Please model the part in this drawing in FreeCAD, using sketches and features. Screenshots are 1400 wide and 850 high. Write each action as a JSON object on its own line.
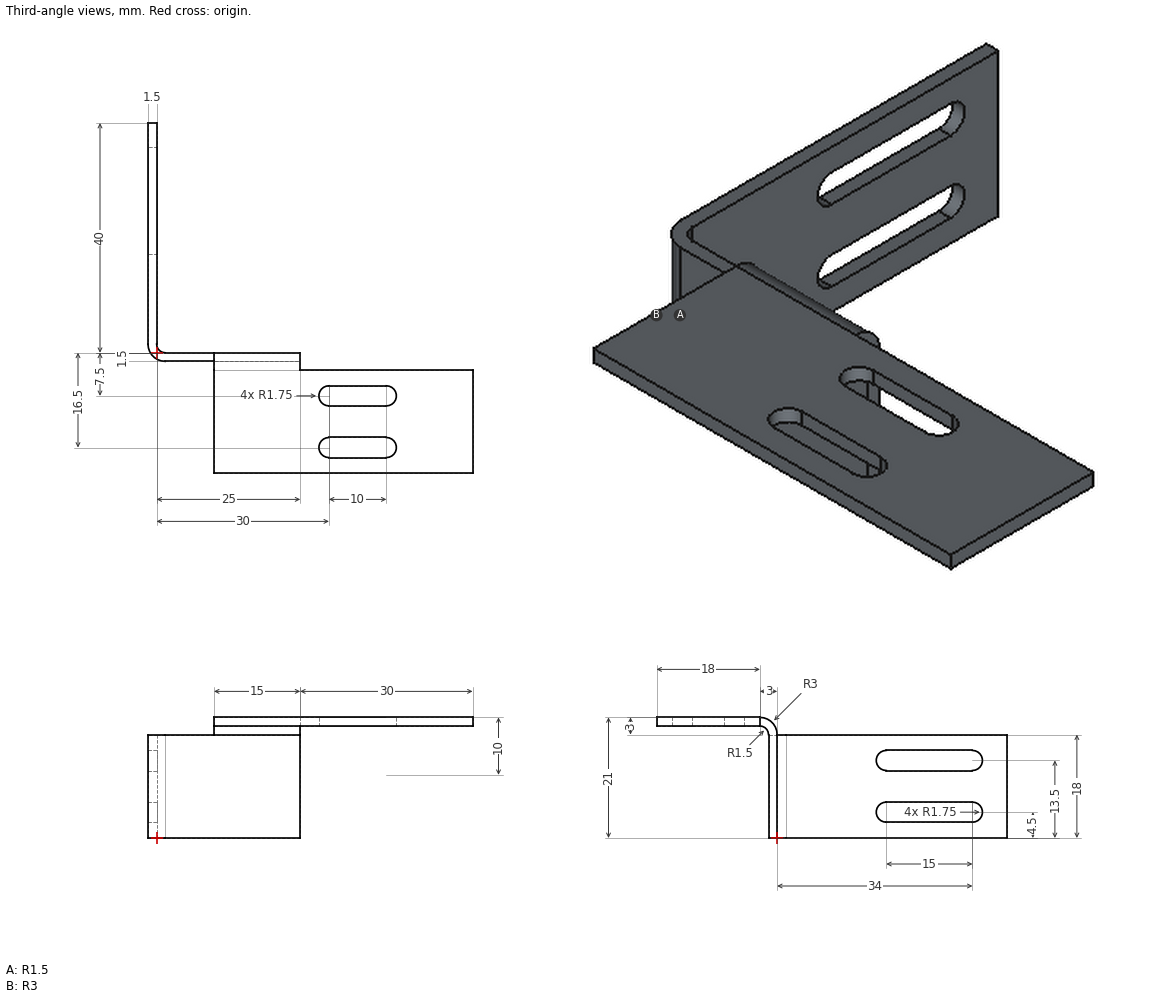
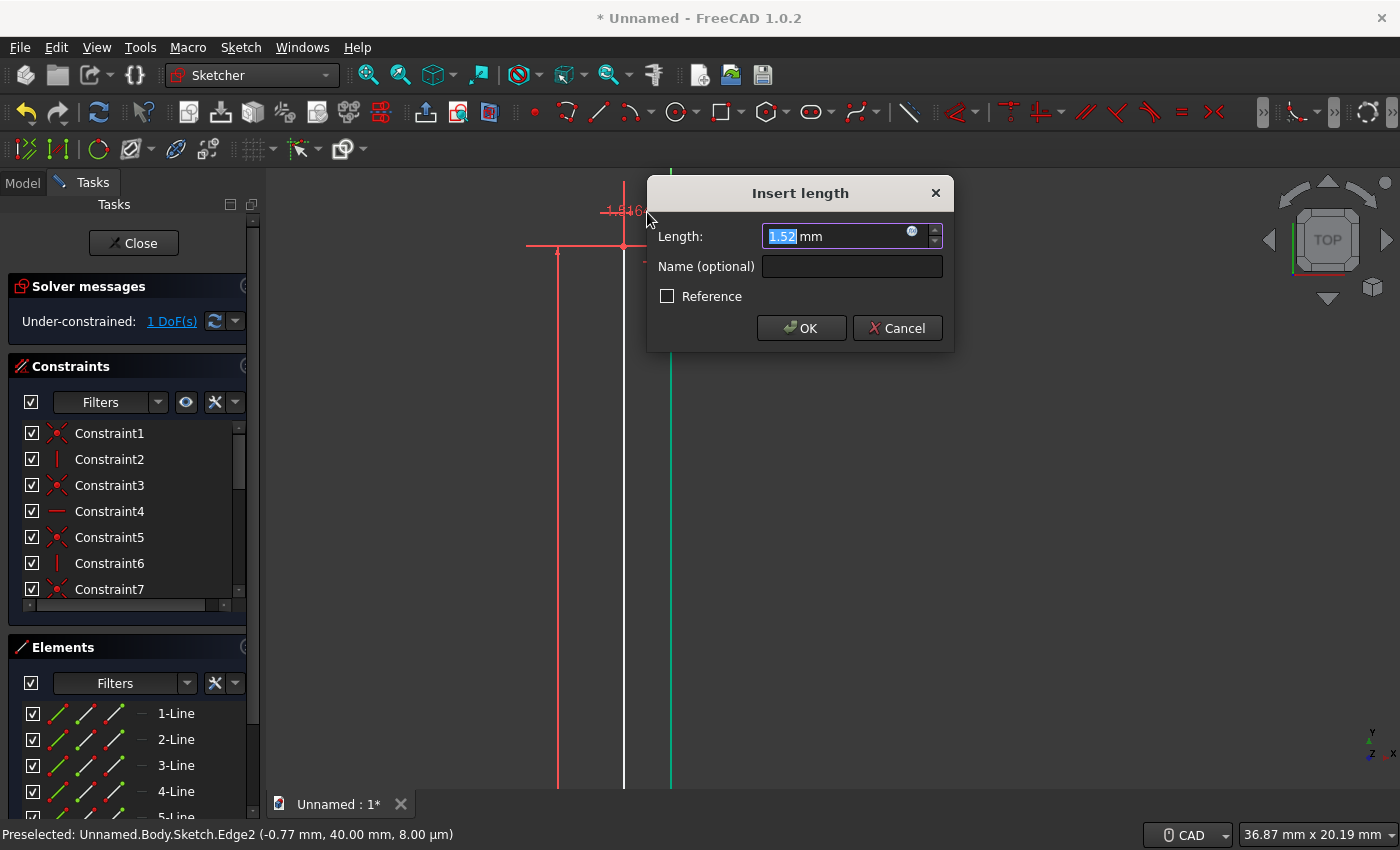
{"action": "type", "text": "1.5"}
{"action": "key", "text": "Return"}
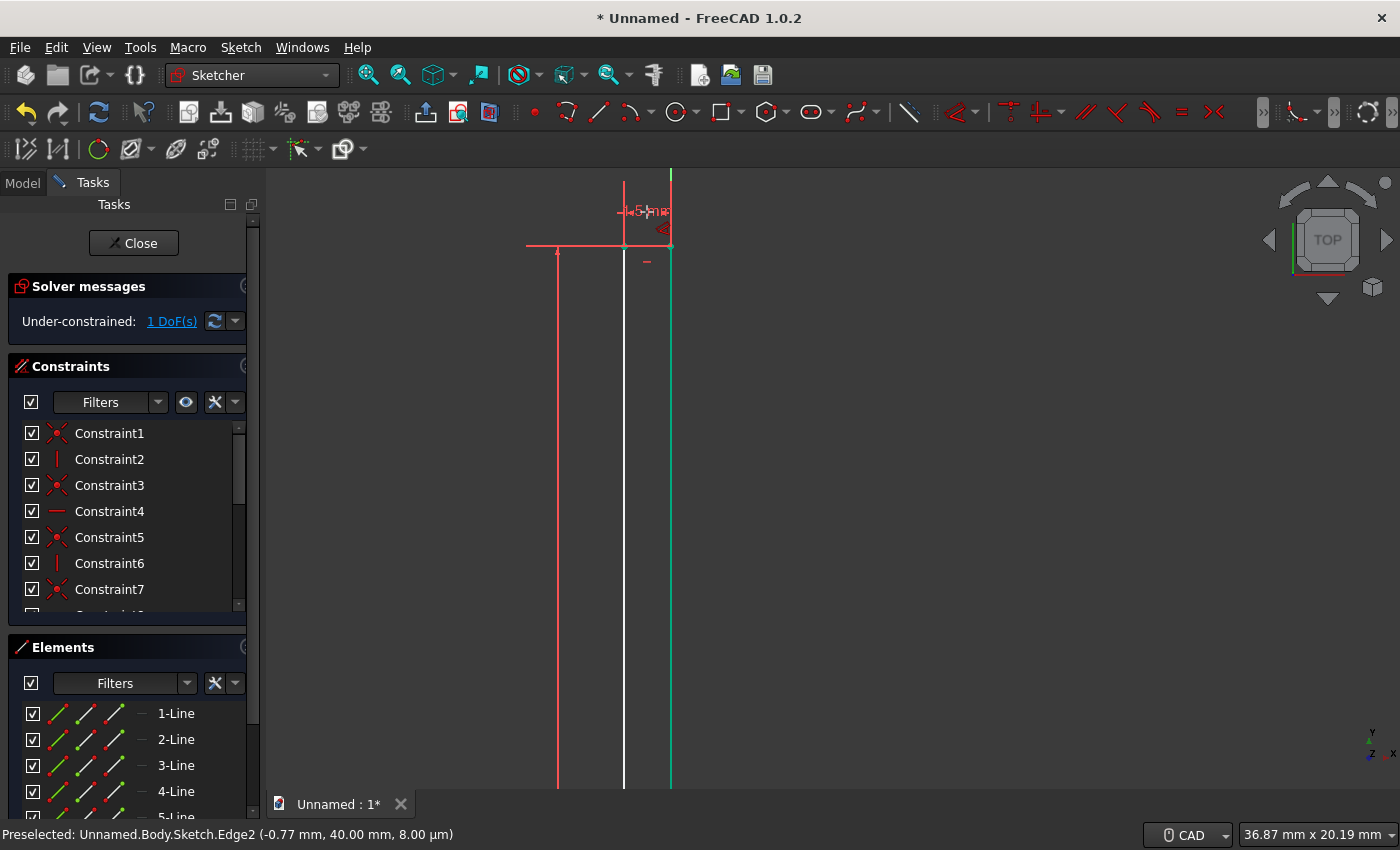
{"action": "scroll", "coordinate": [649, 304], "scroll_direction": "down", "scroll_amount": 6}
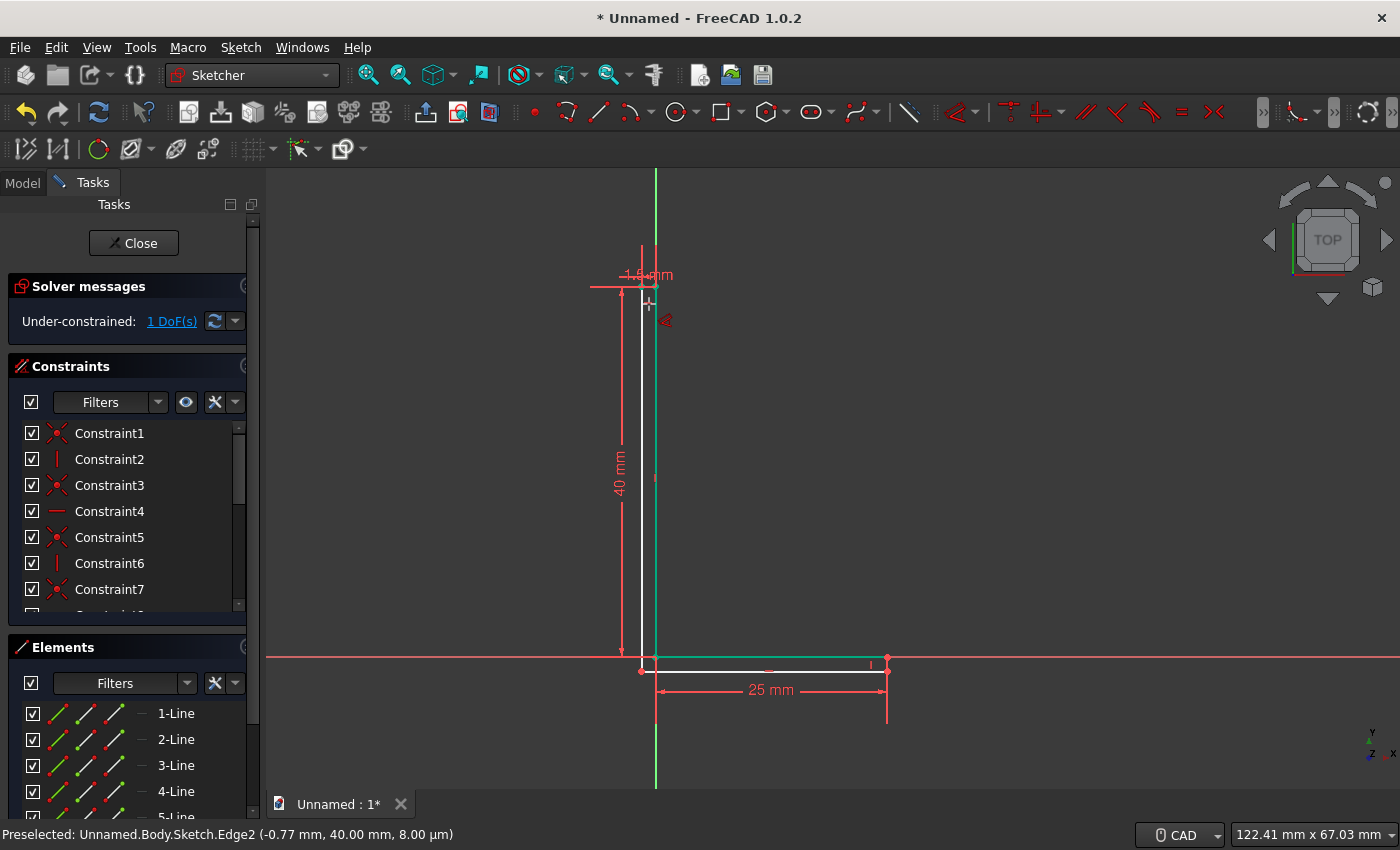
{"action": "scroll", "coordinate": [887, 668], "scroll_direction": "up", "scroll_amount": 6}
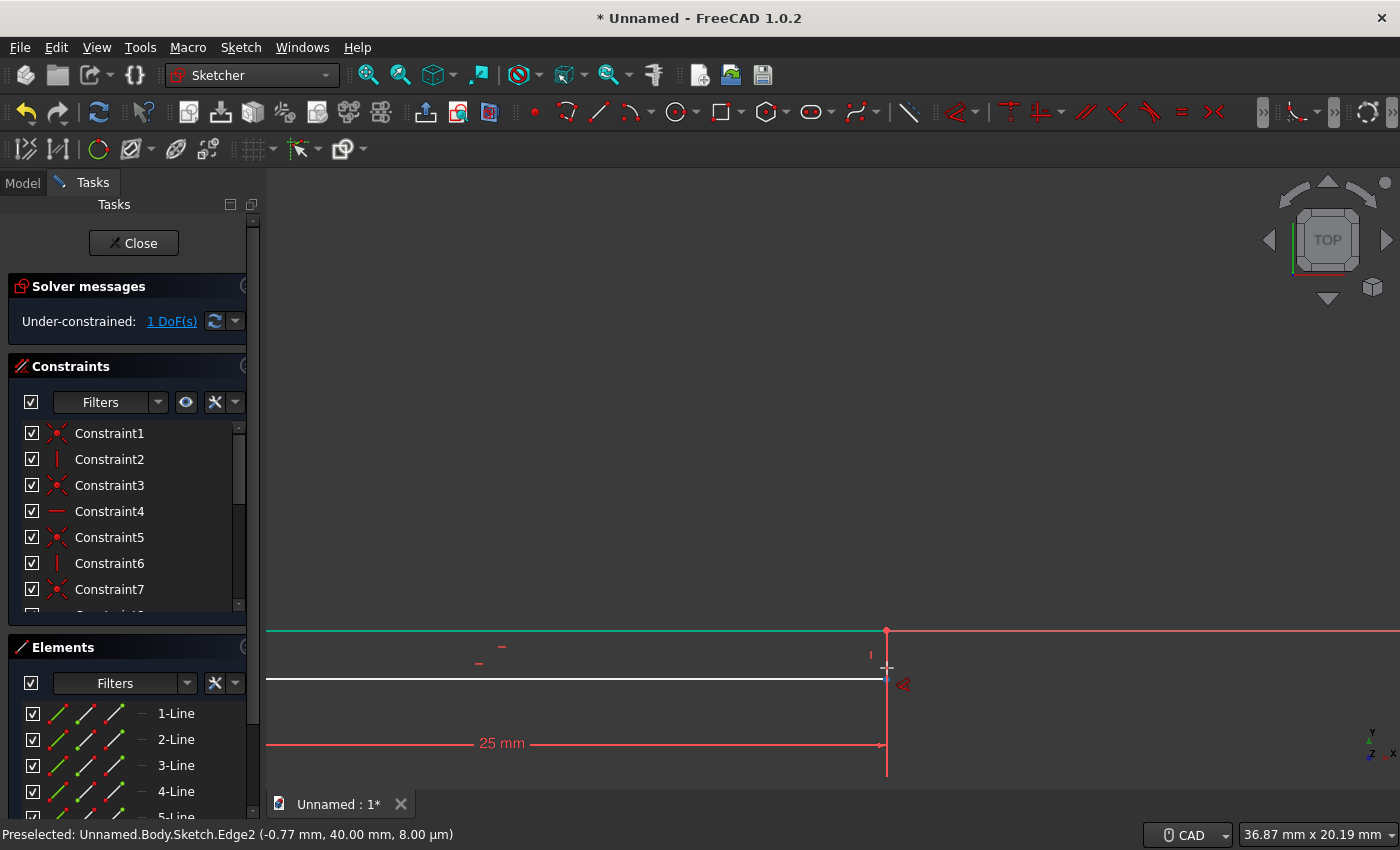
{"action": "left_click", "coordinate": [887, 665]}
{"action": "left_click", "coordinate": [921, 655]}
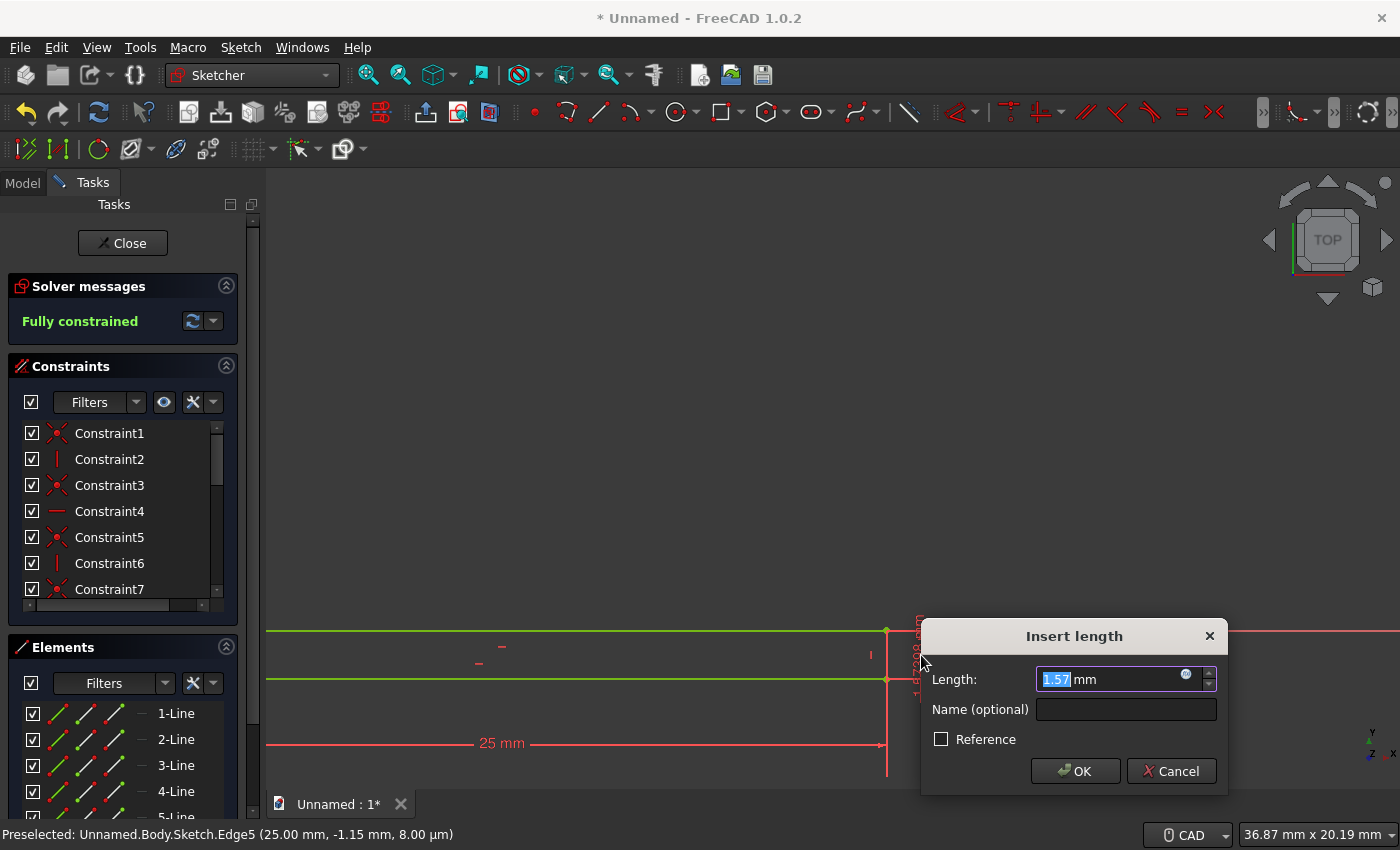
{"action": "type", "text": "1.5"}
{"action": "key", "text": "Return"}
{"action": "key", "text": "Escape"}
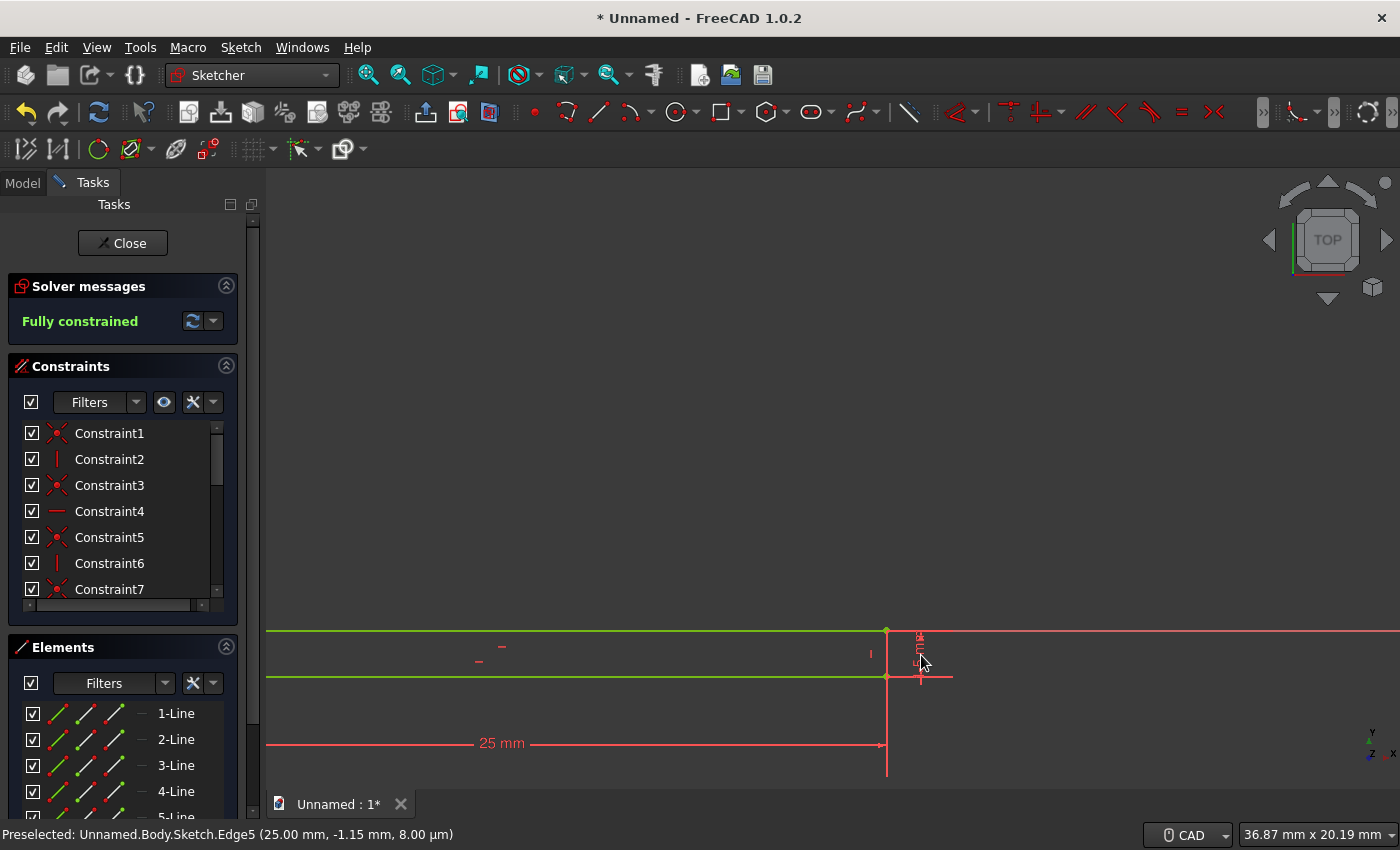
{"action": "left_click", "coordinate": [123, 243]}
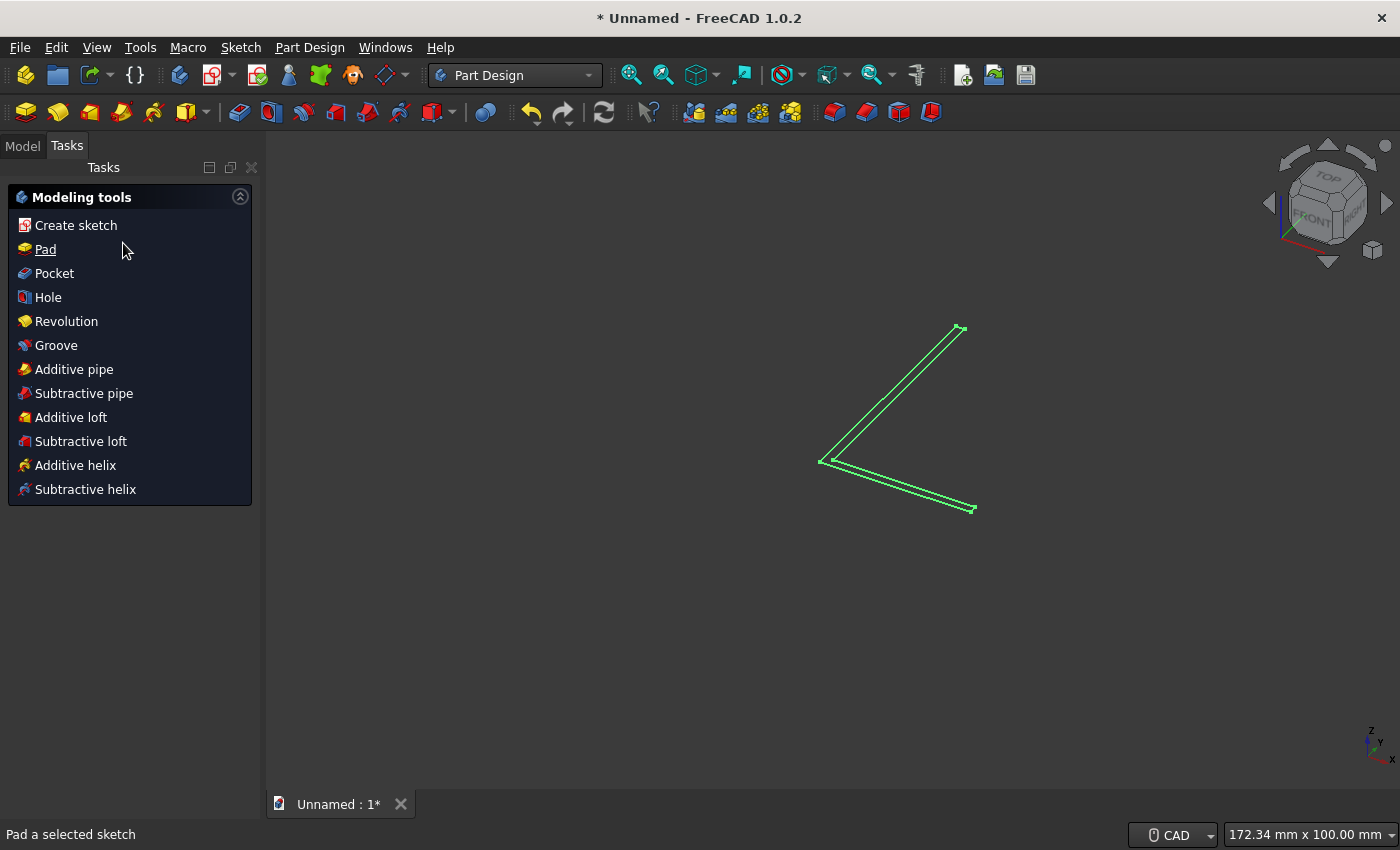
{"action": "left_click", "coordinate": [26, 112]}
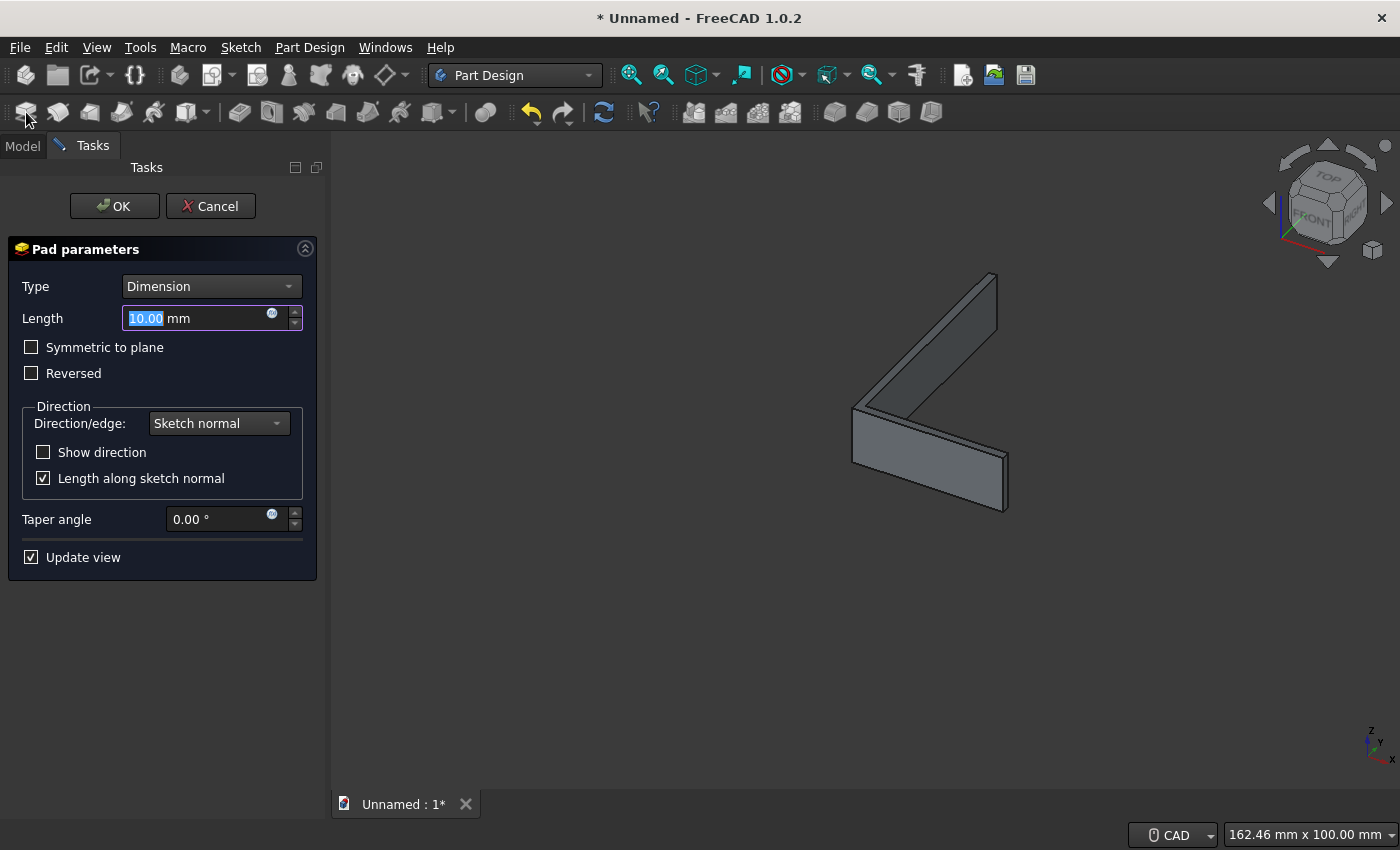
{"action": "type", "text": "18"}
{"action": "key", "text": "Tab"}